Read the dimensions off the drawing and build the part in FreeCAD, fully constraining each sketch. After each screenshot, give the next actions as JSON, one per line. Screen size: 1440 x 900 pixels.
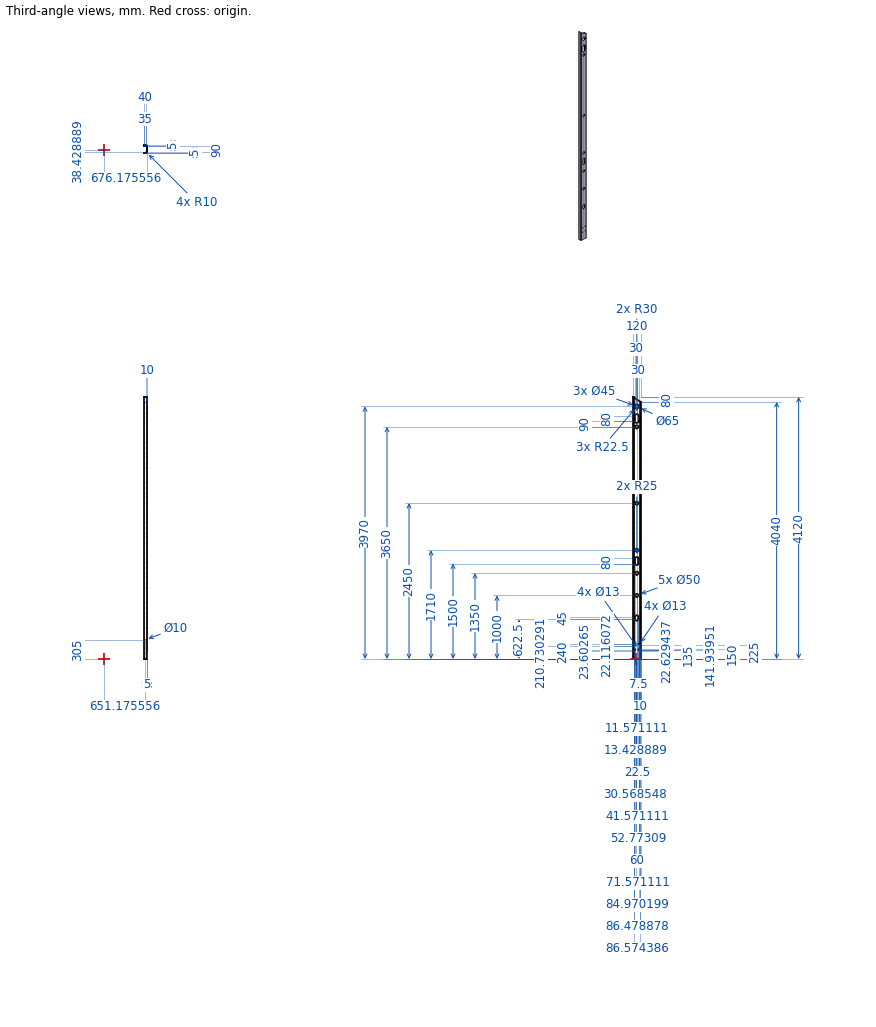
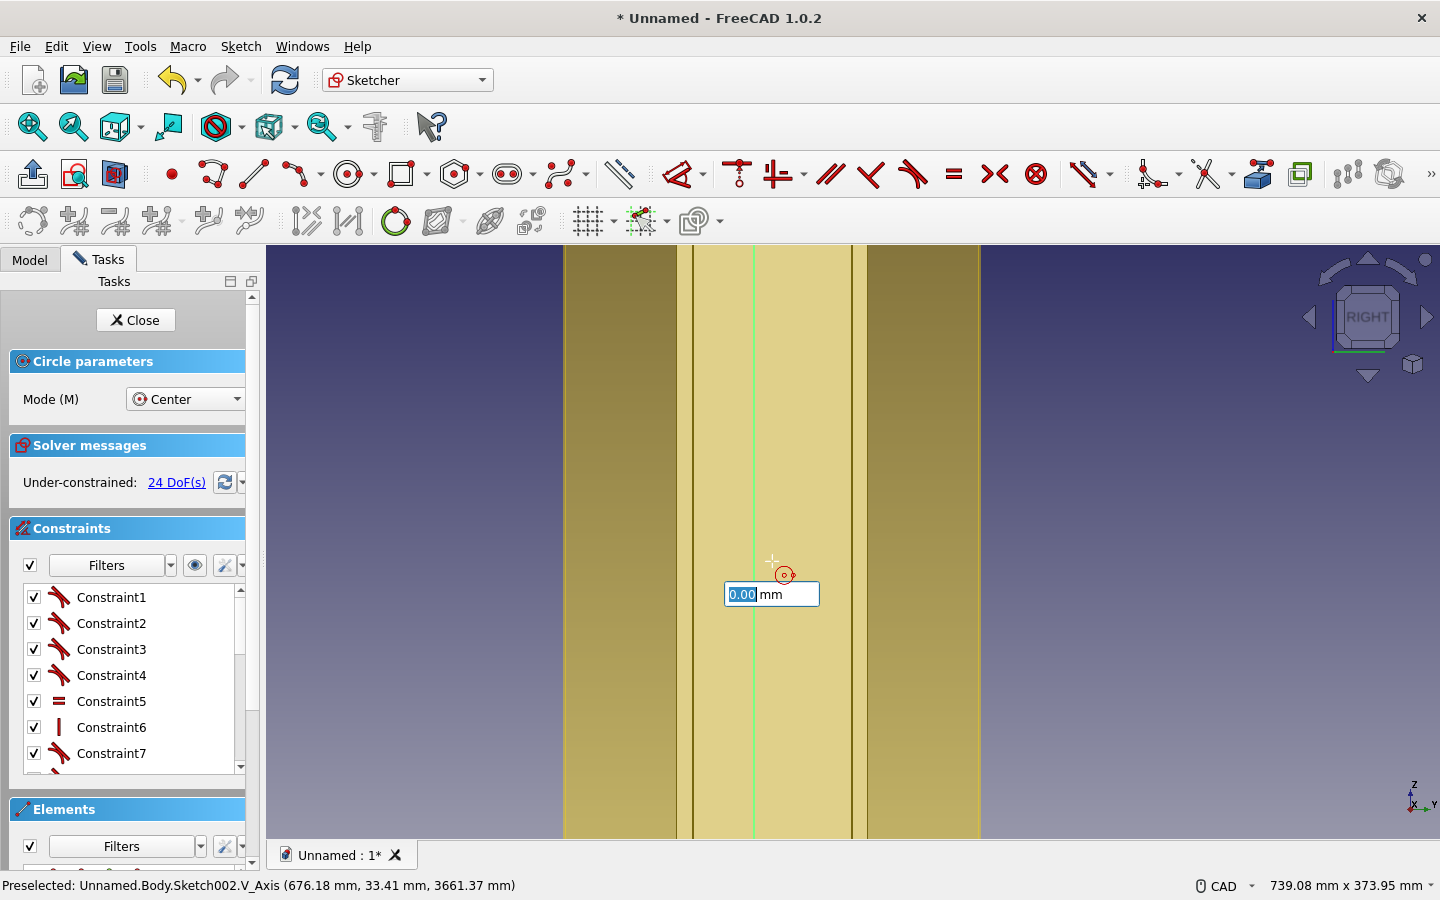
{"action": "scroll", "coordinate": [785, 570], "scroll_direction": "down", "scroll_amount": 14}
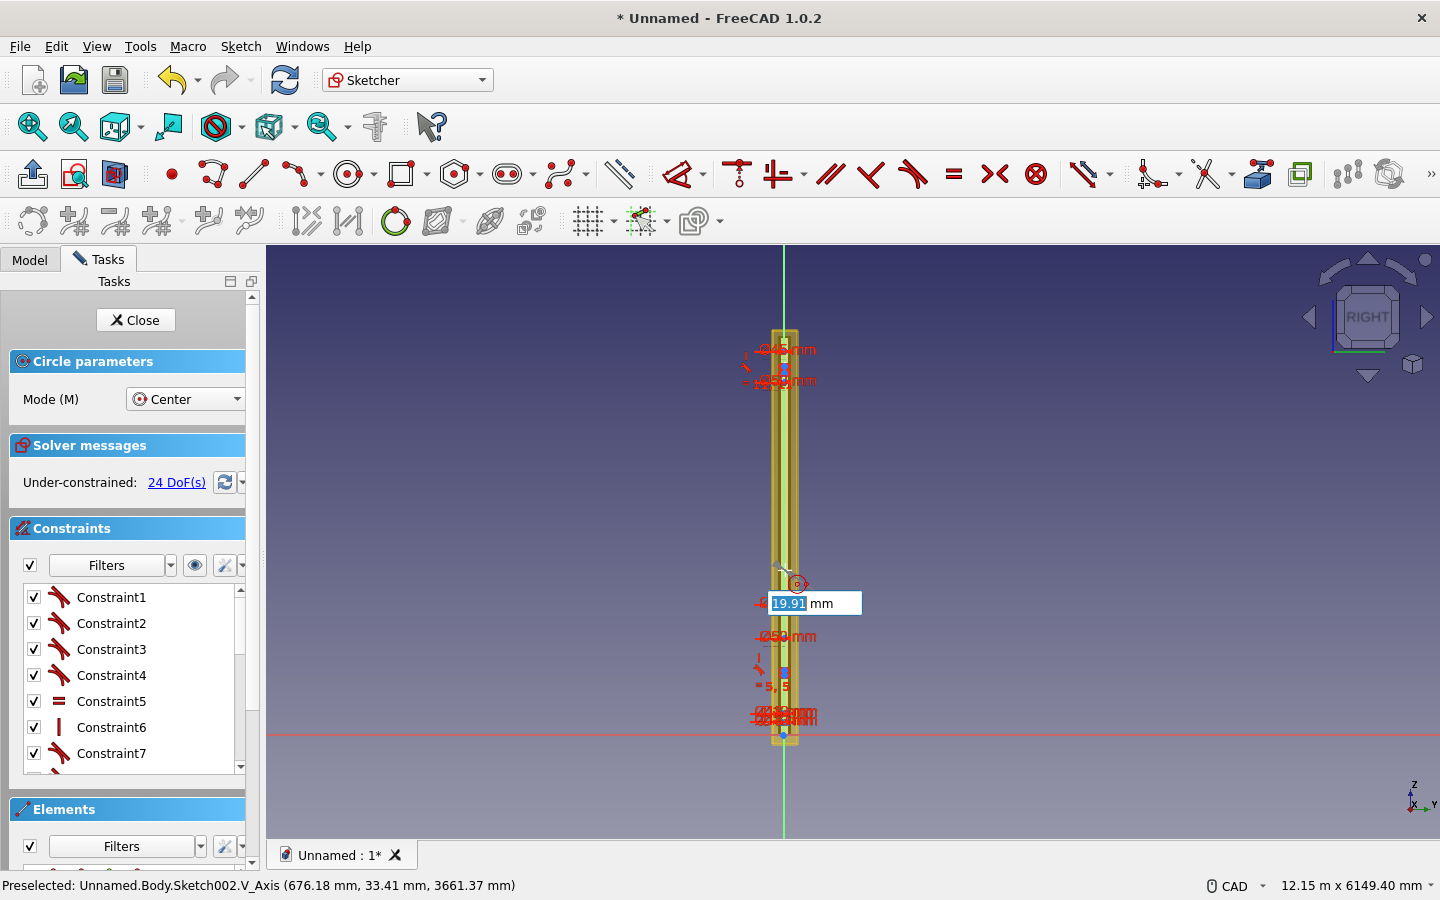
{"action": "scroll", "coordinate": [786, 568], "scroll_direction": "up", "scroll_amount": 9}
{"action": "mouse_move", "coordinate": [786, 567]}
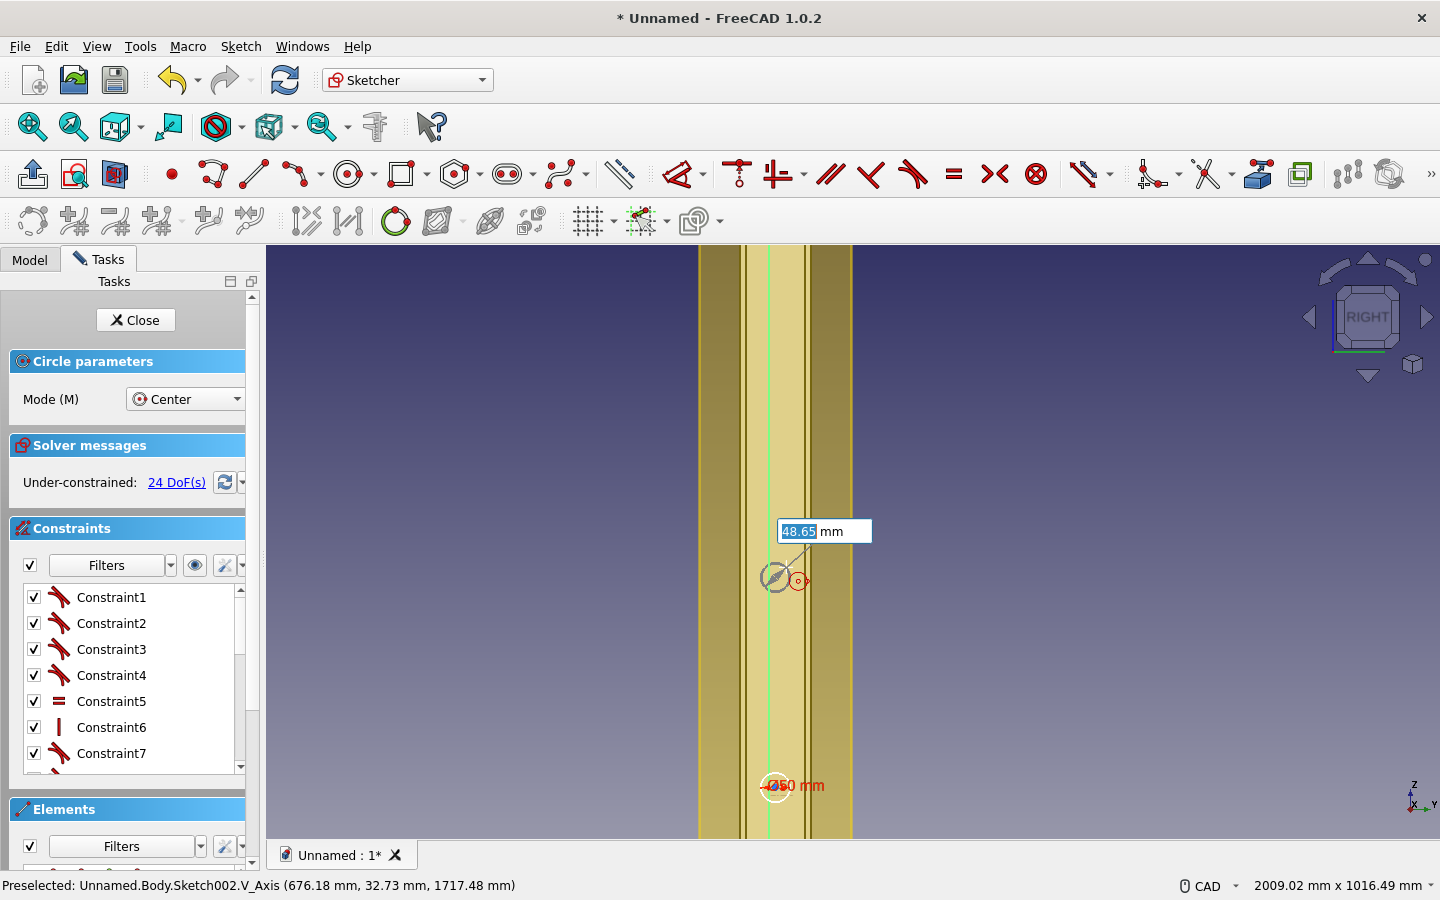
{"action": "type", "text": "50"}
{"action": "key", "text": "Return"}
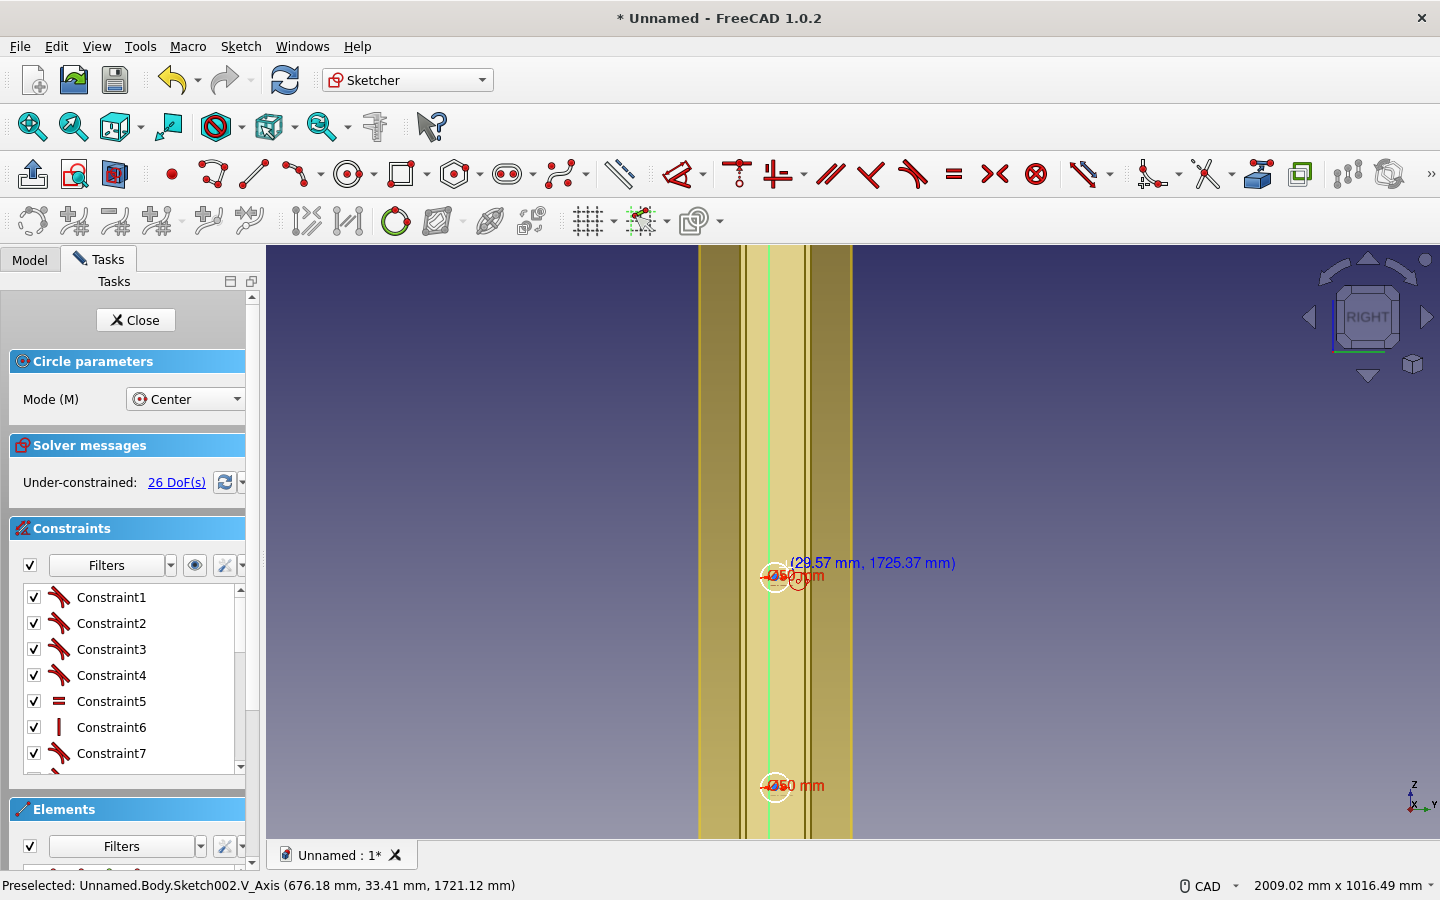
{"action": "scroll", "coordinate": [786, 568], "scroll_direction": "down", "scroll_amount": 9}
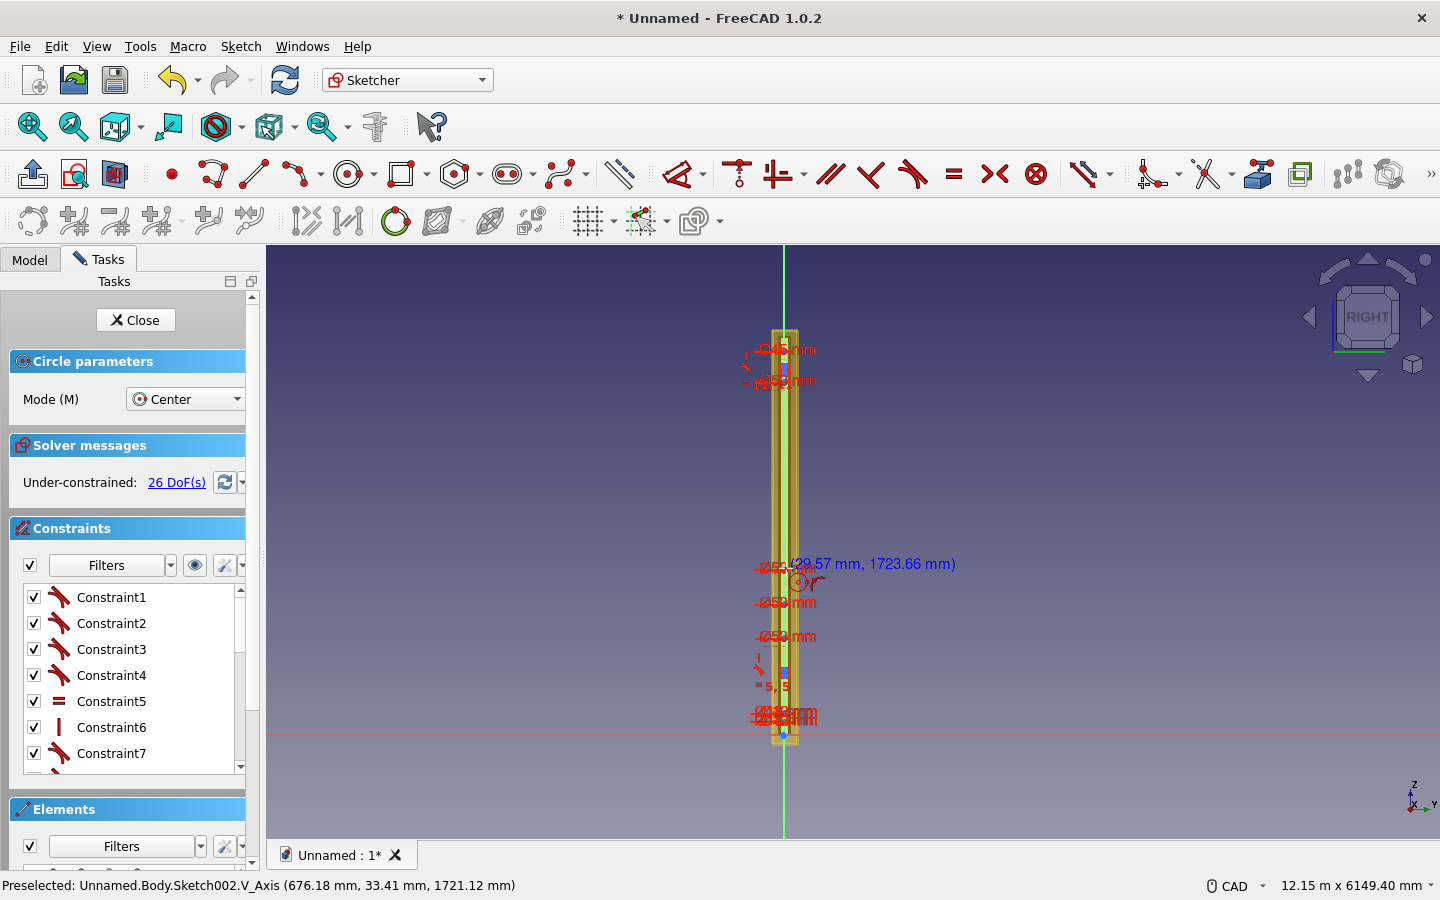
{"action": "scroll", "coordinate": [785, 498], "scroll_direction": "up", "scroll_amount": 14}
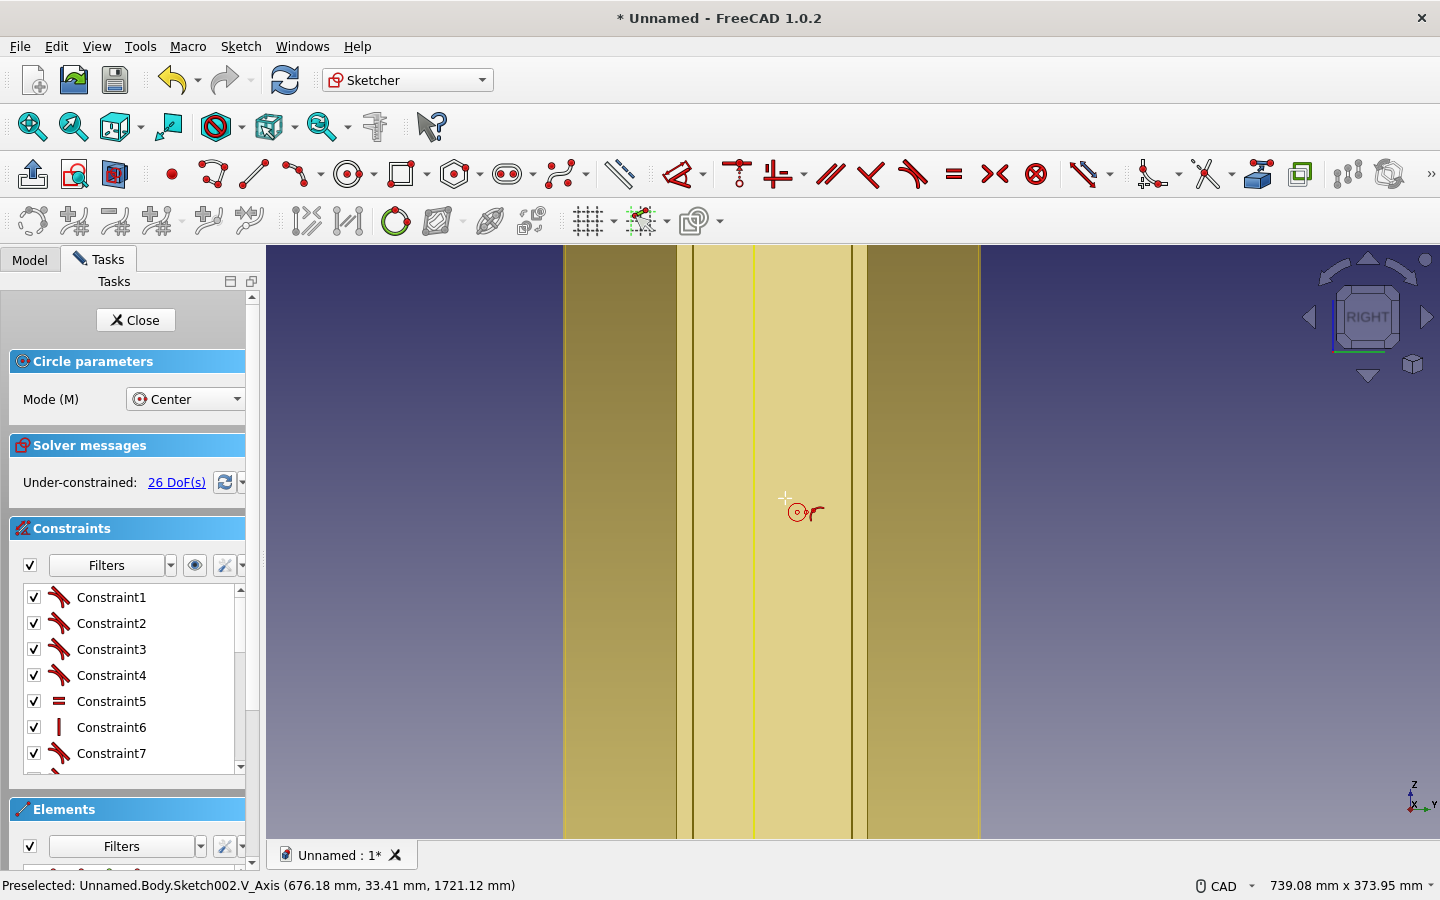
{"action": "left_click", "coordinate": [772, 499]}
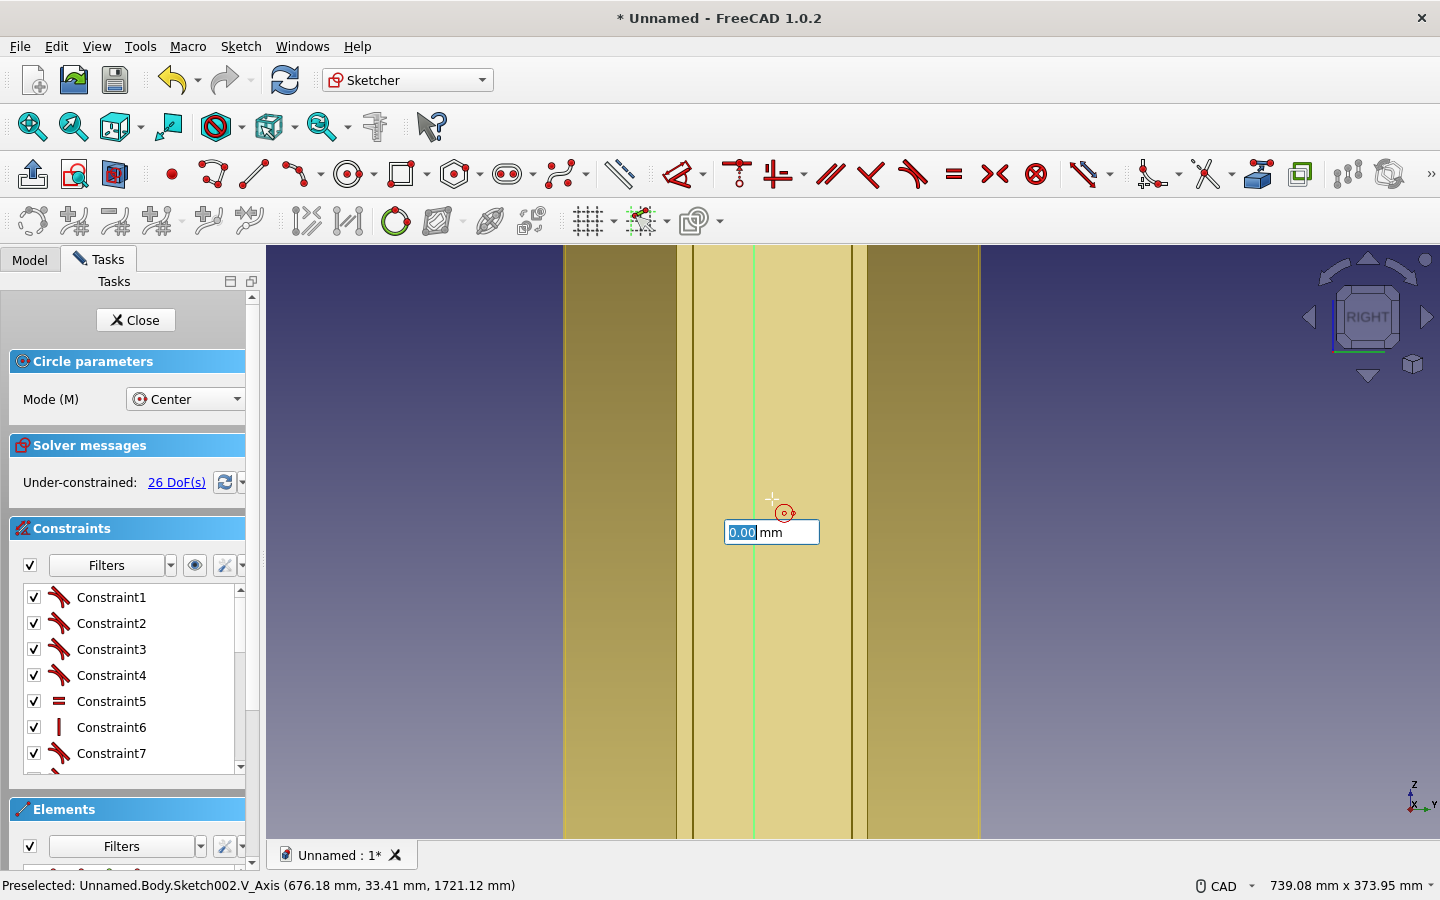
{"action": "scroll", "coordinate": [785, 498], "scroll_direction": "down", "scroll_amount": 14}